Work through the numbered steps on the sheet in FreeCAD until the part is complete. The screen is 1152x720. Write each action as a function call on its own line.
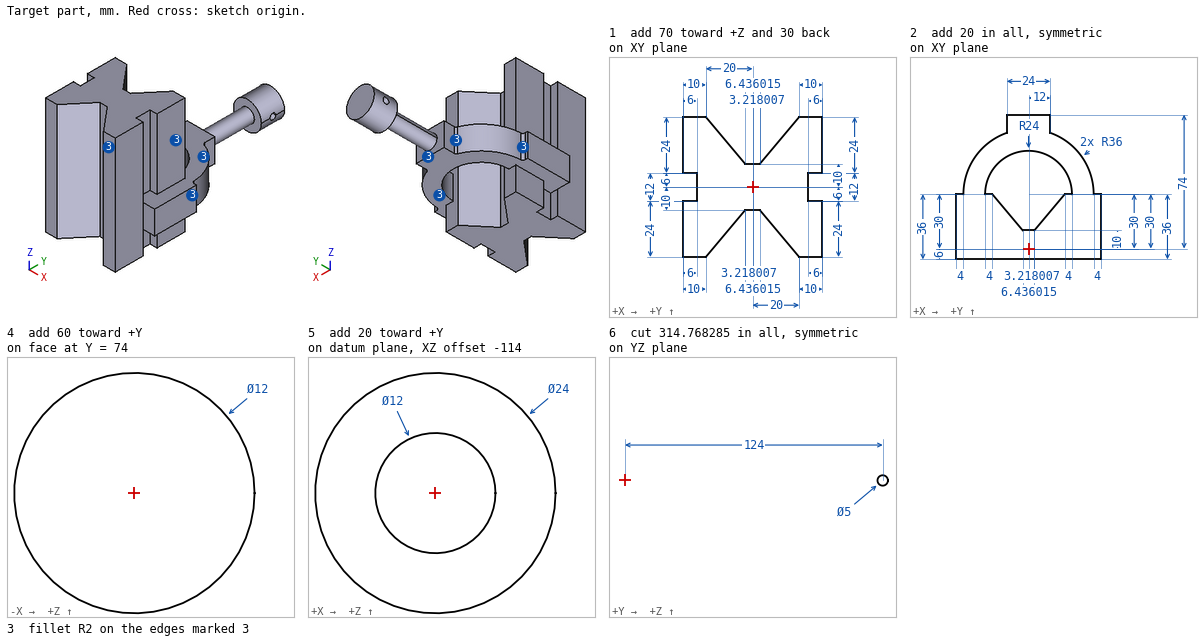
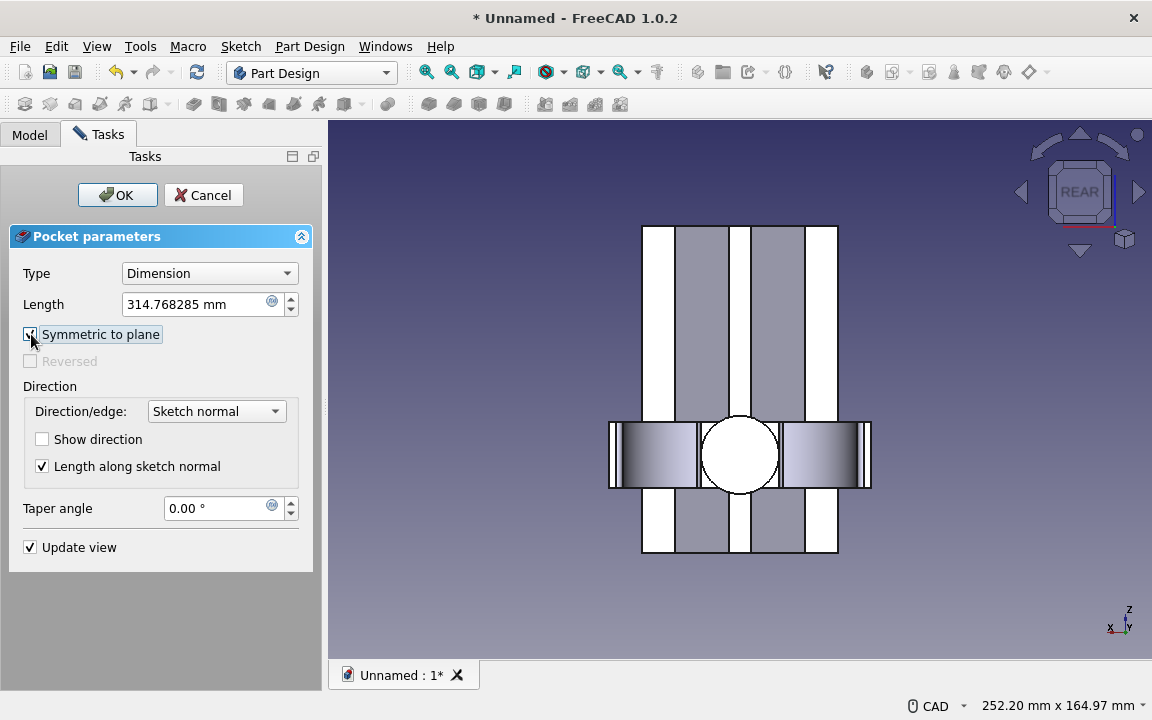
click(118, 195)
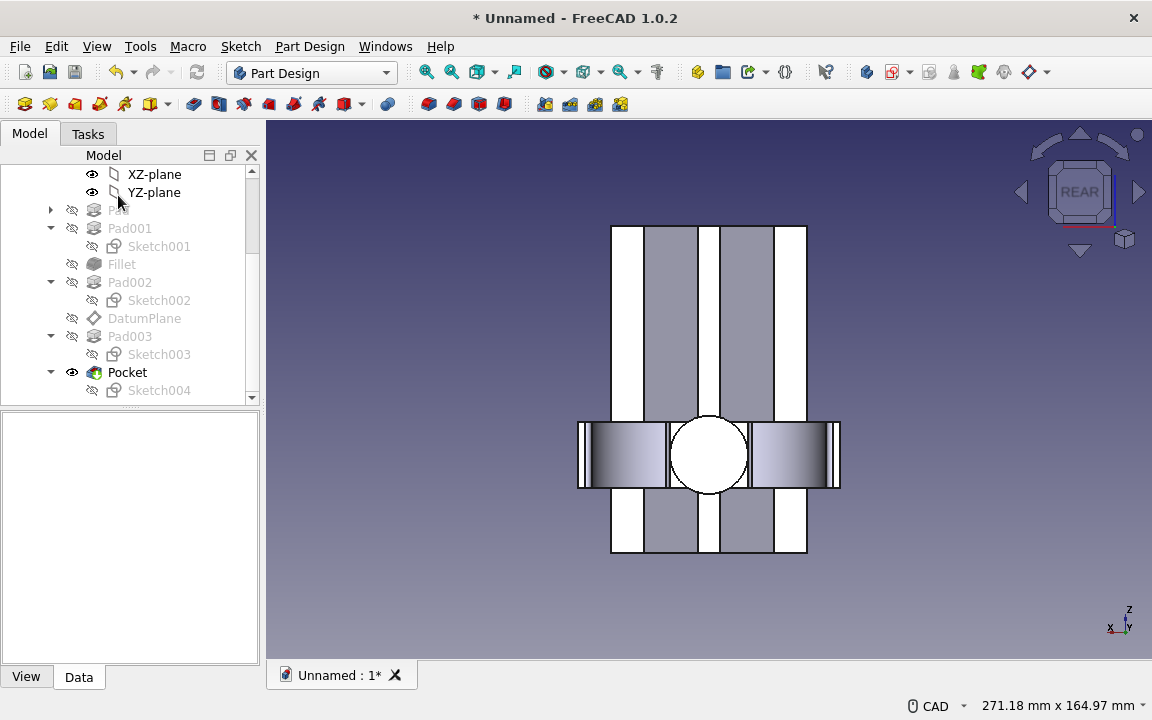
key(0)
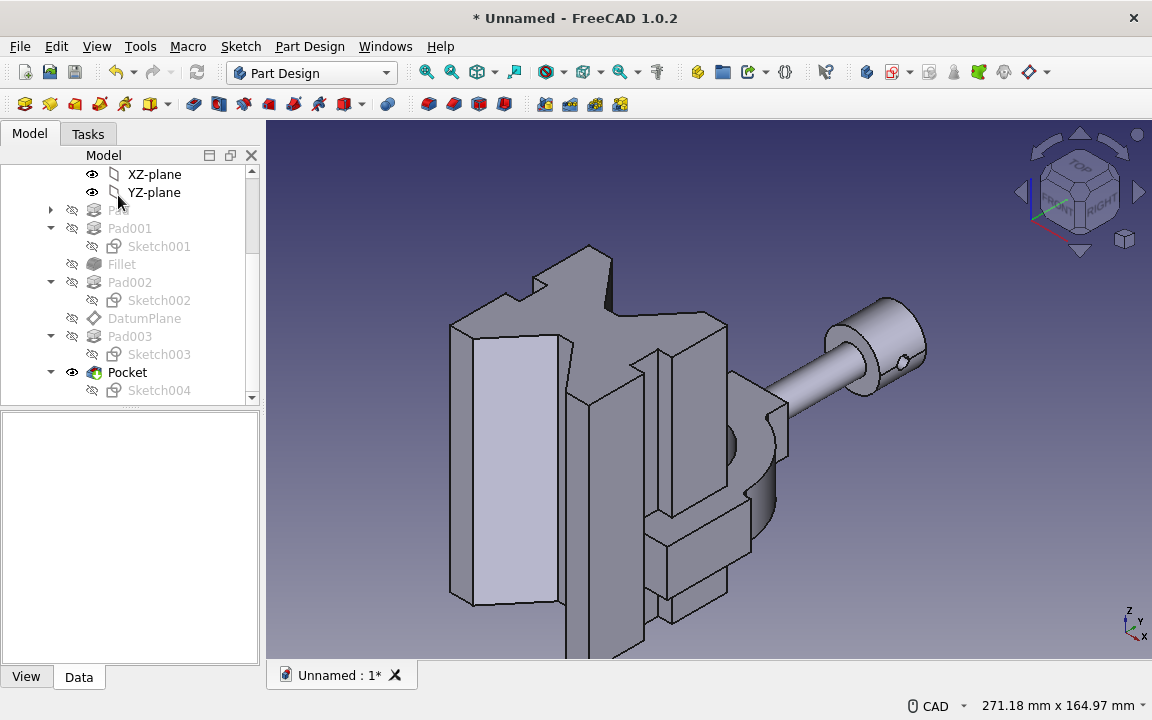
click(427, 72)